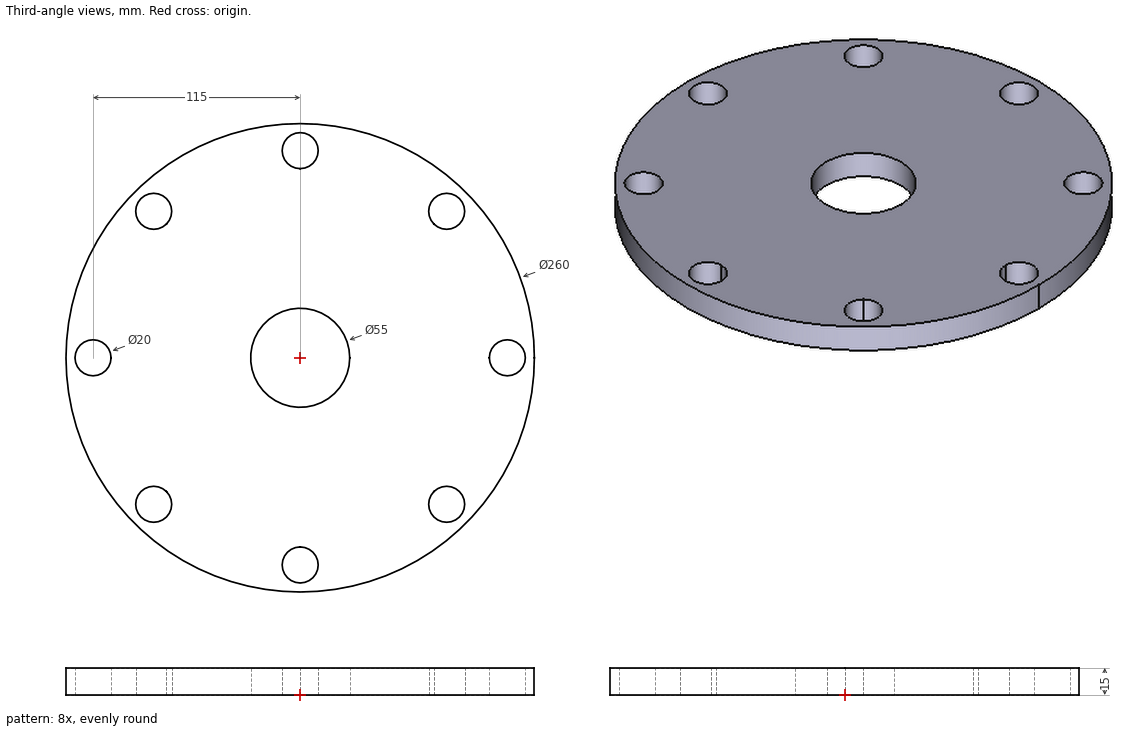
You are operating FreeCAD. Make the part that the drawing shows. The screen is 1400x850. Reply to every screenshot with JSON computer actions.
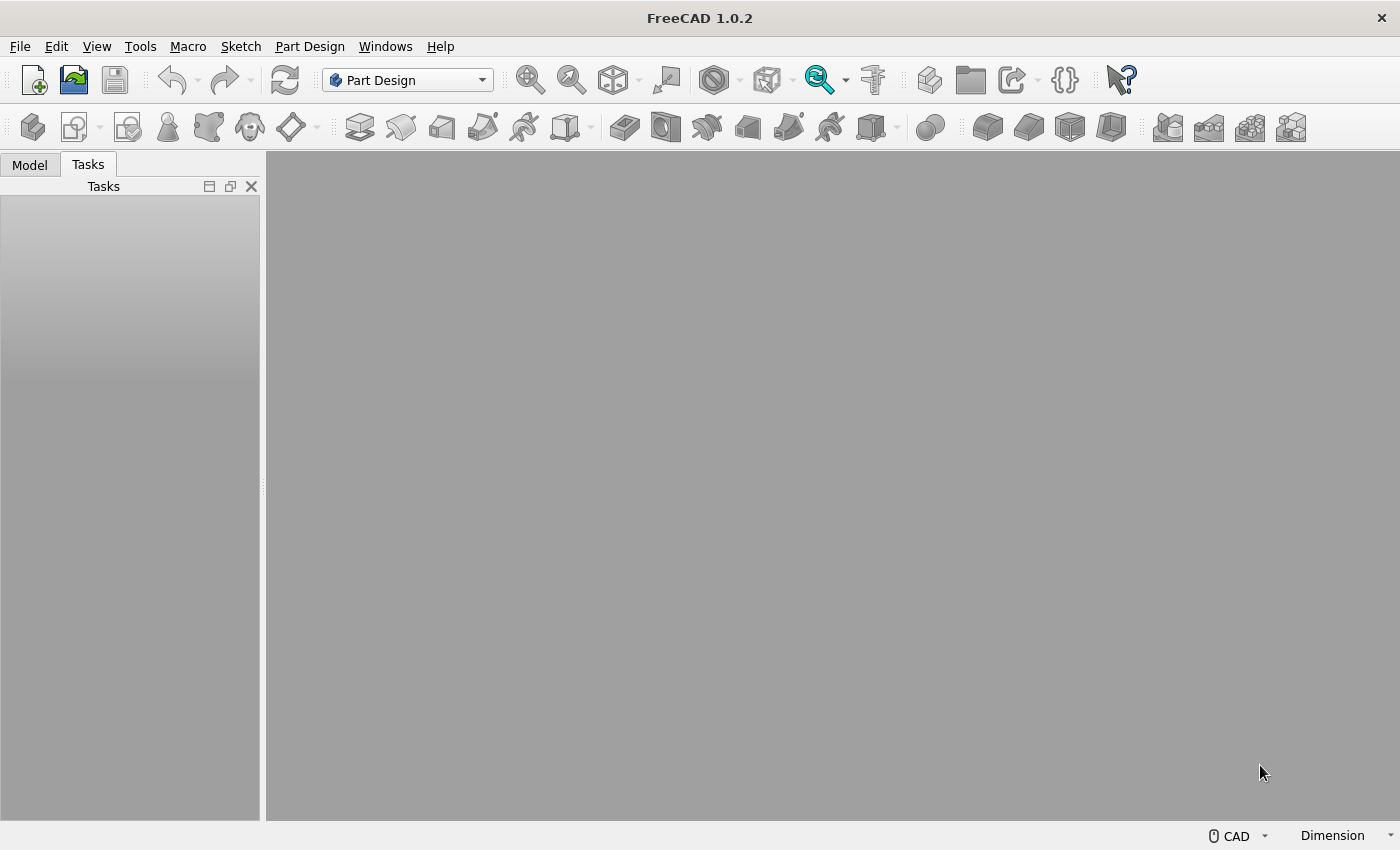
{"action": "left_click", "coordinate": [33, 80]}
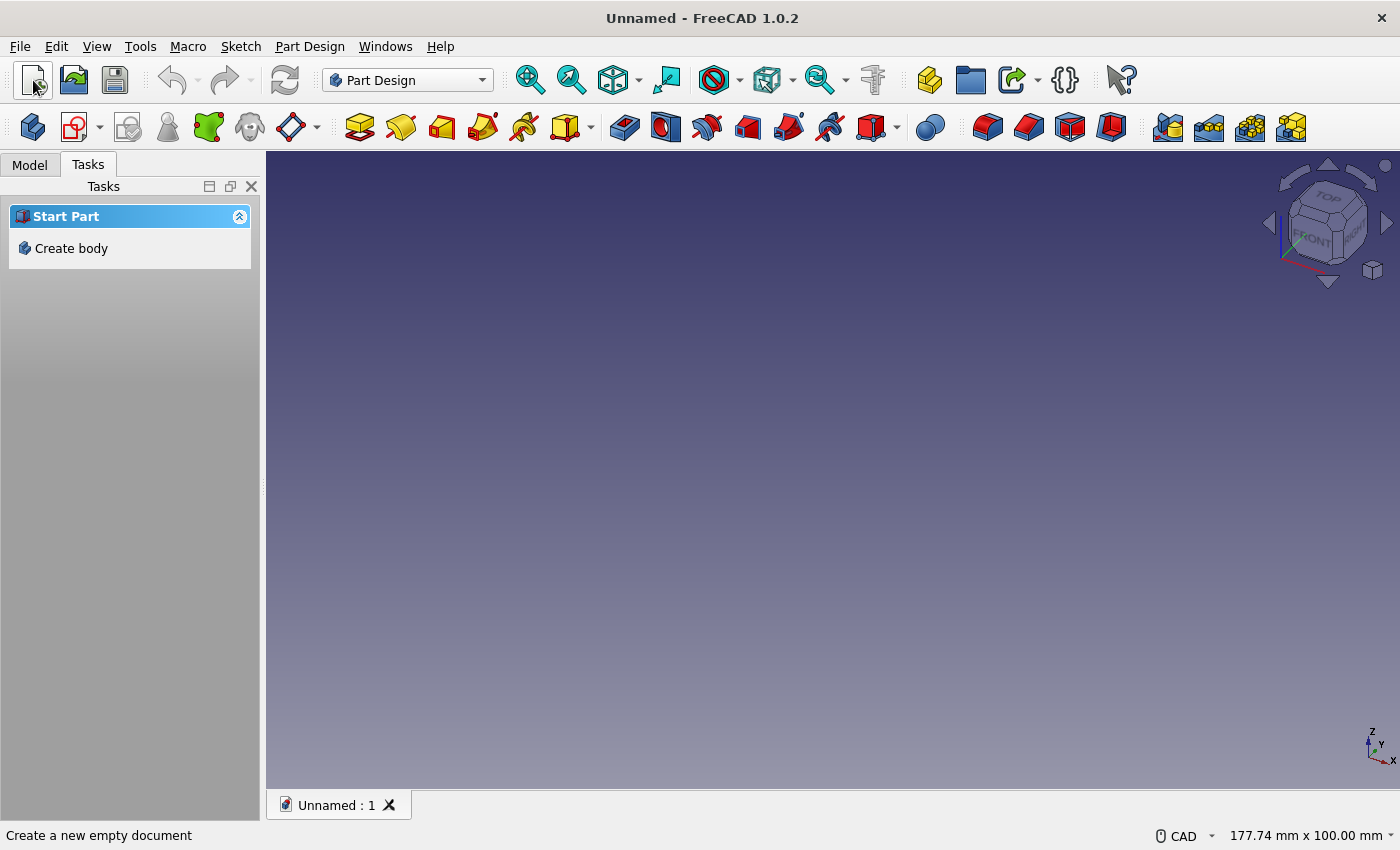
{"action": "left_click", "coordinate": [74, 128]}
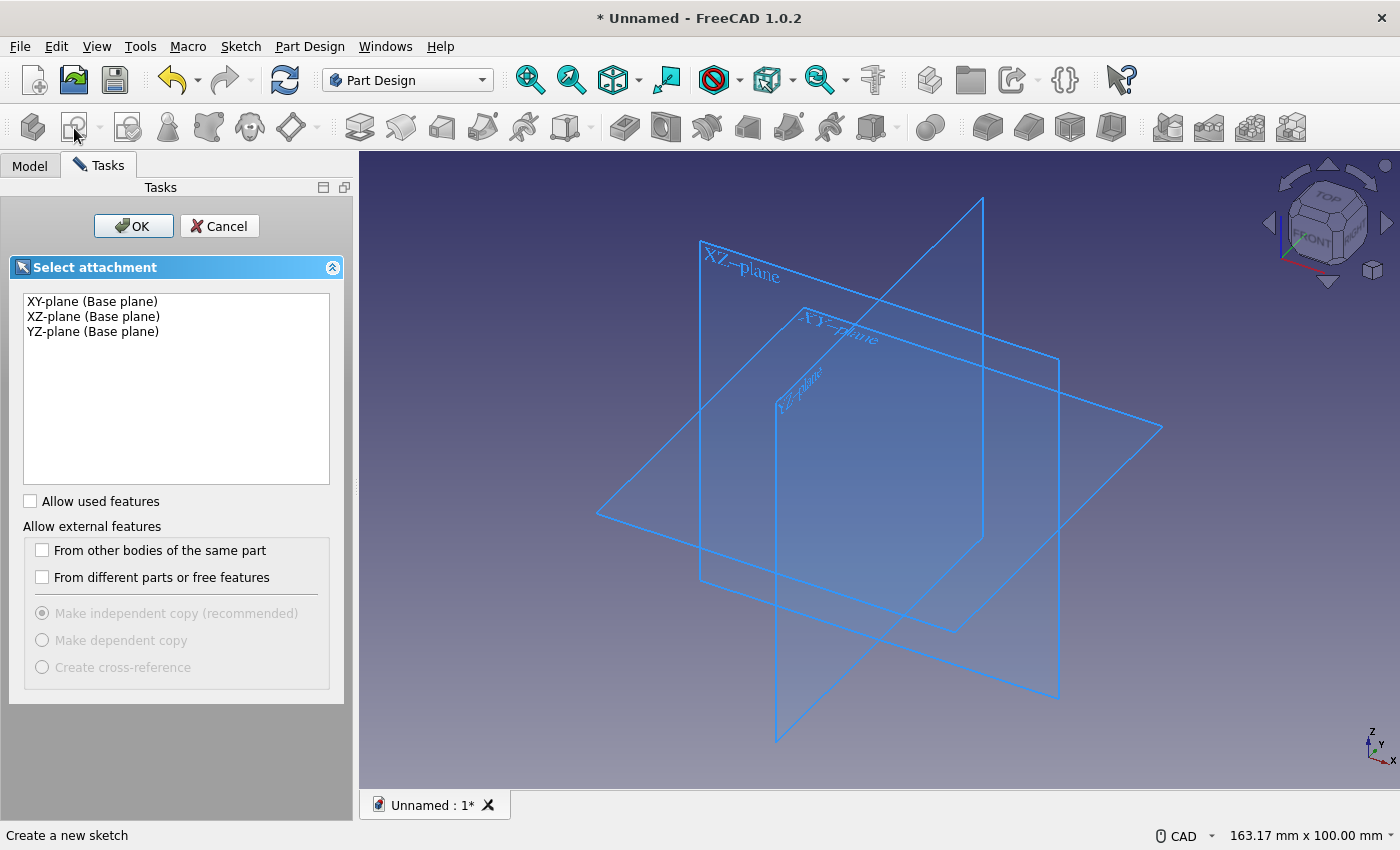
{"action": "left_click", "coordinate": [84, 302]}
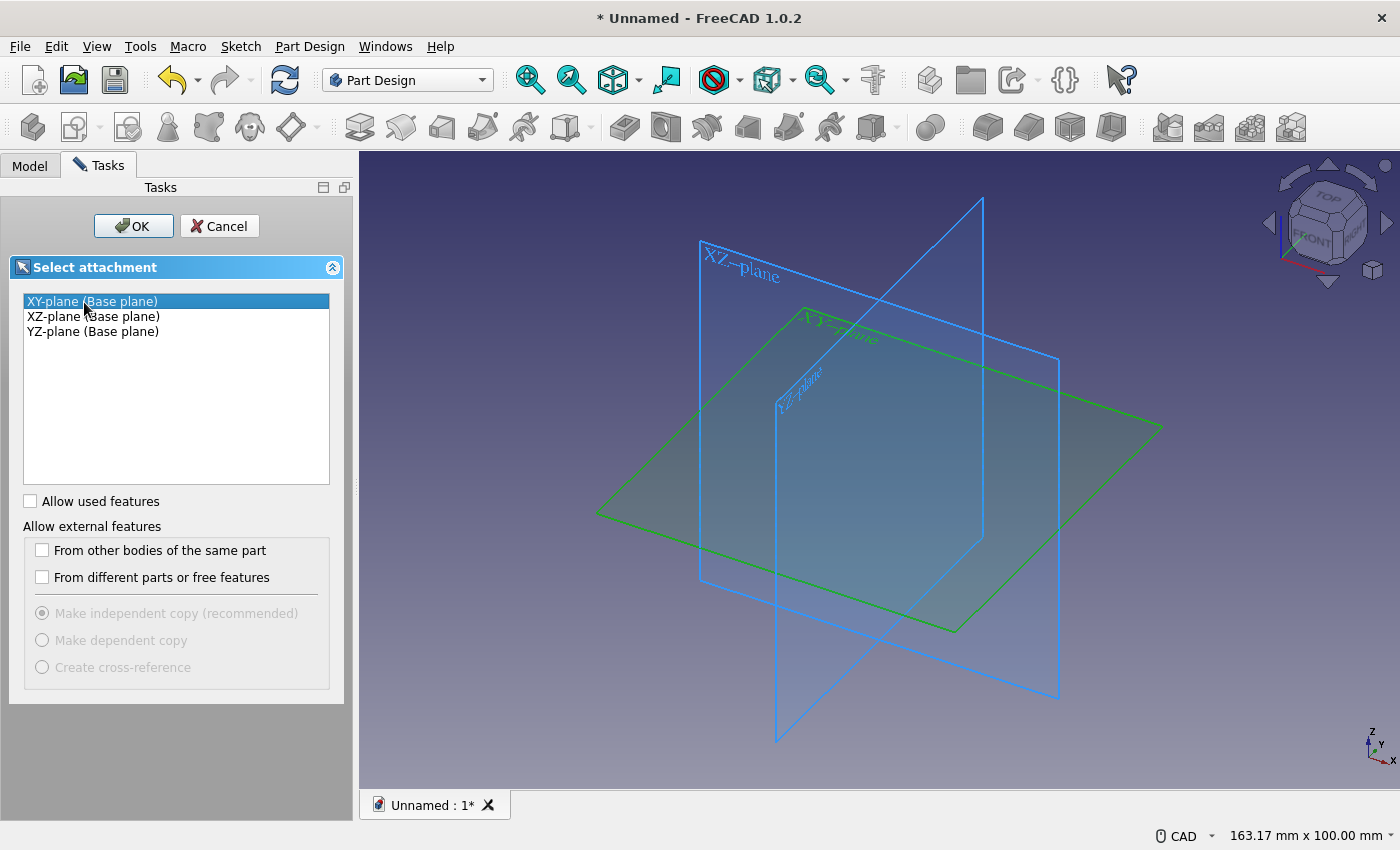
{"action": "left_click", "coordinate": [134, 226]}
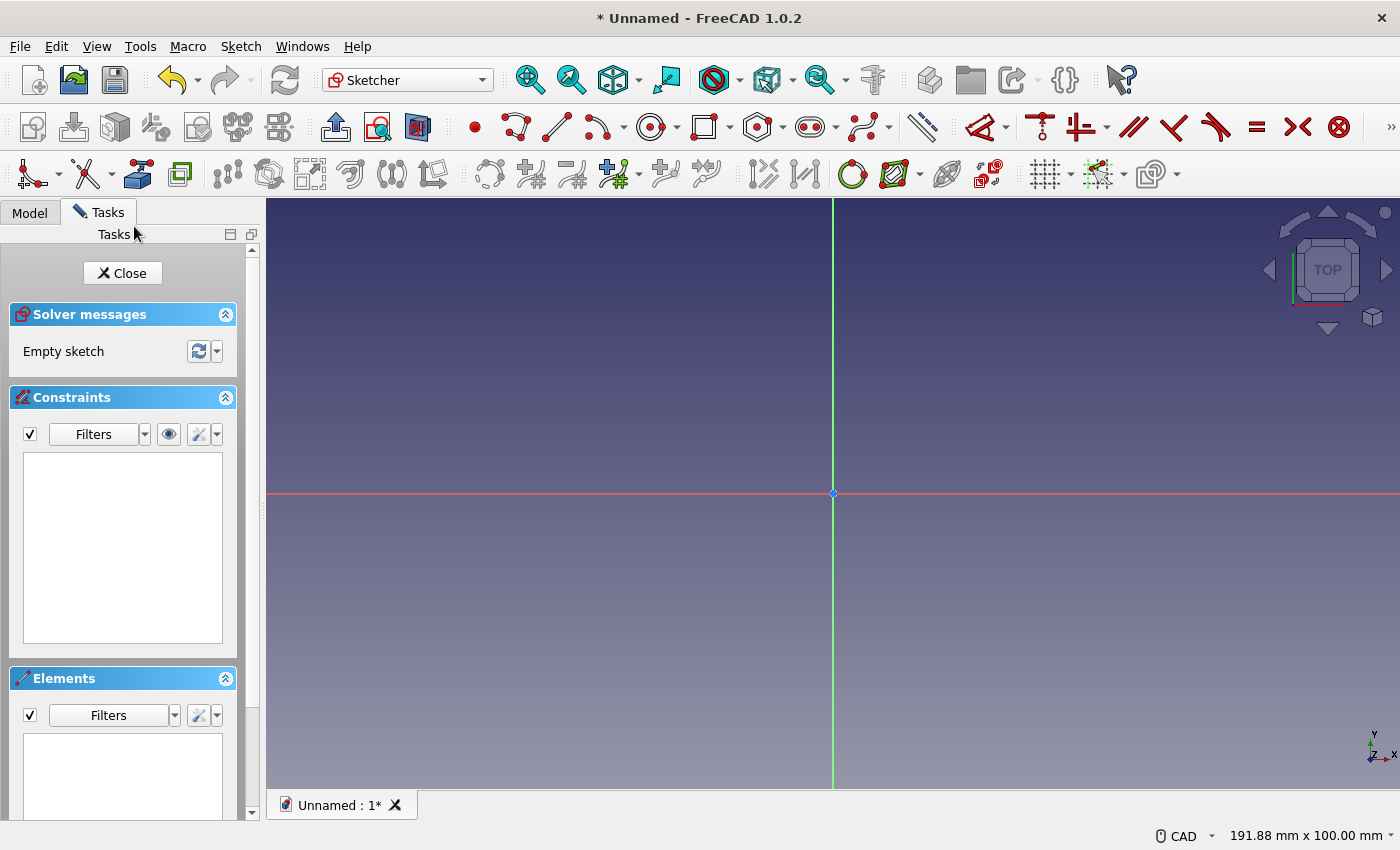
{"action": "scroll", "coordinate": [742, 494], "scroll_direction": "down", "scroll_amount": 7}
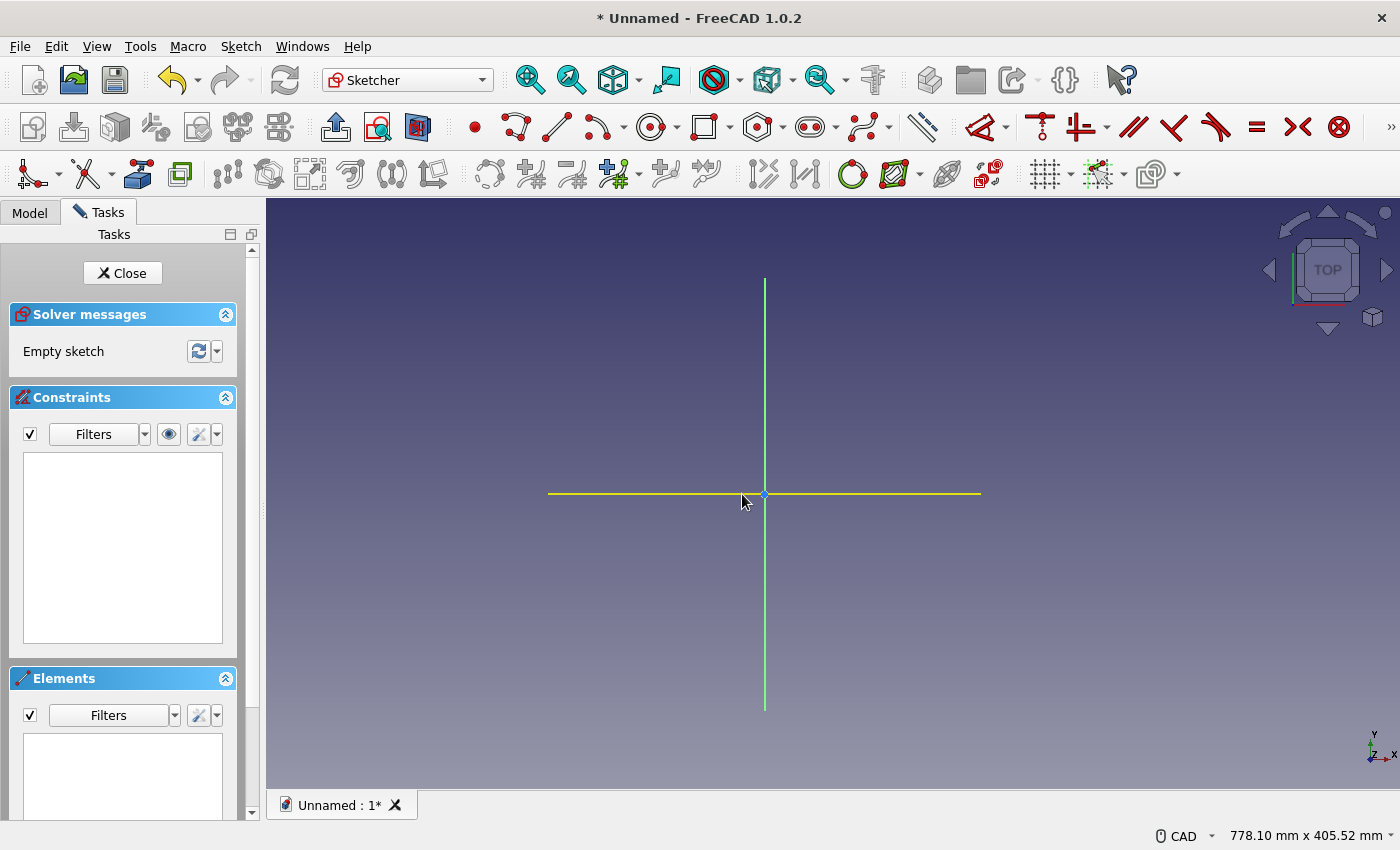
{"action": "left_click", "coordinate": [650, 128]}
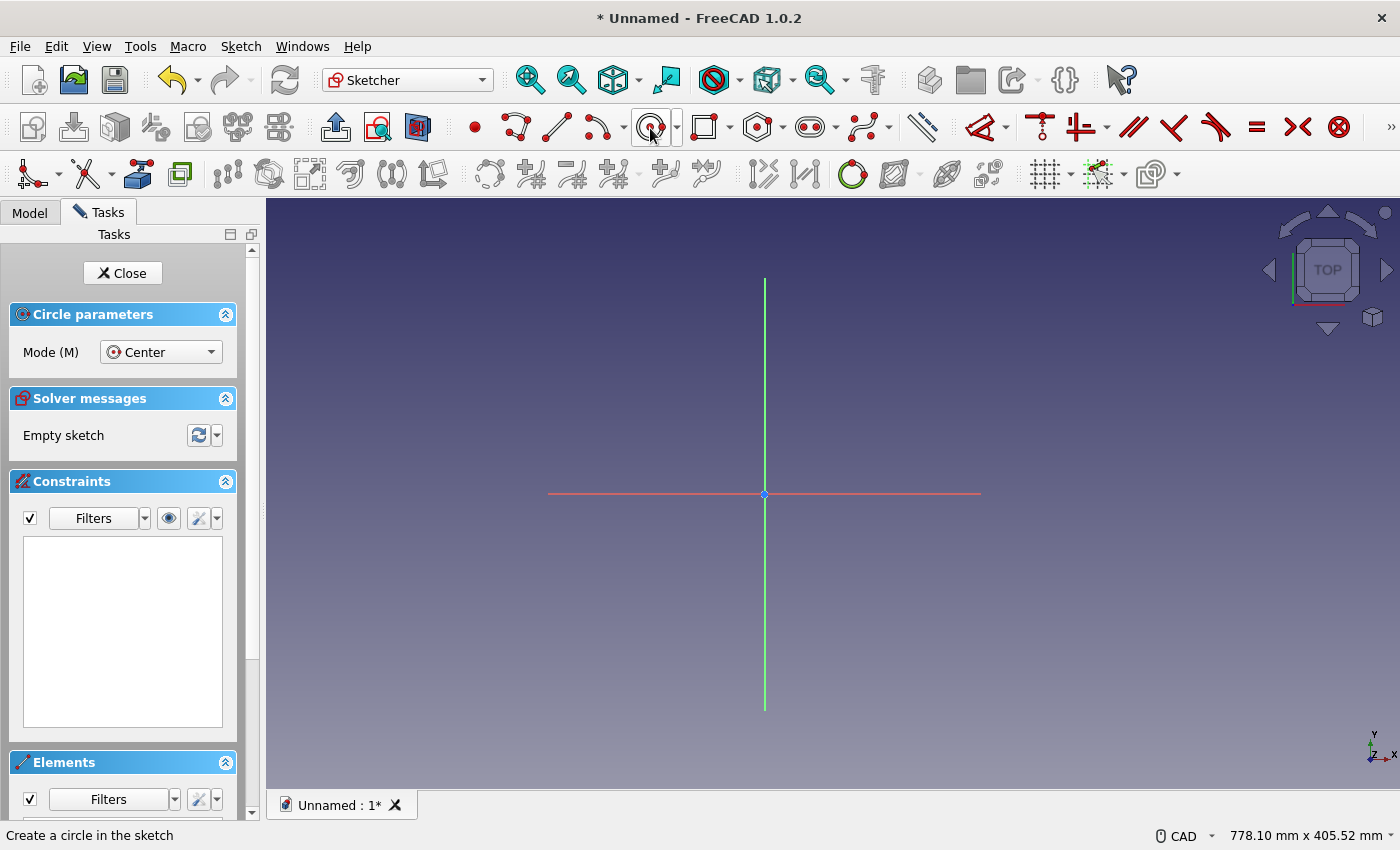
{"action": "left_click", "coordinate": [765, 494]}
{"action": "left_click", "coordinate": [899, 360]}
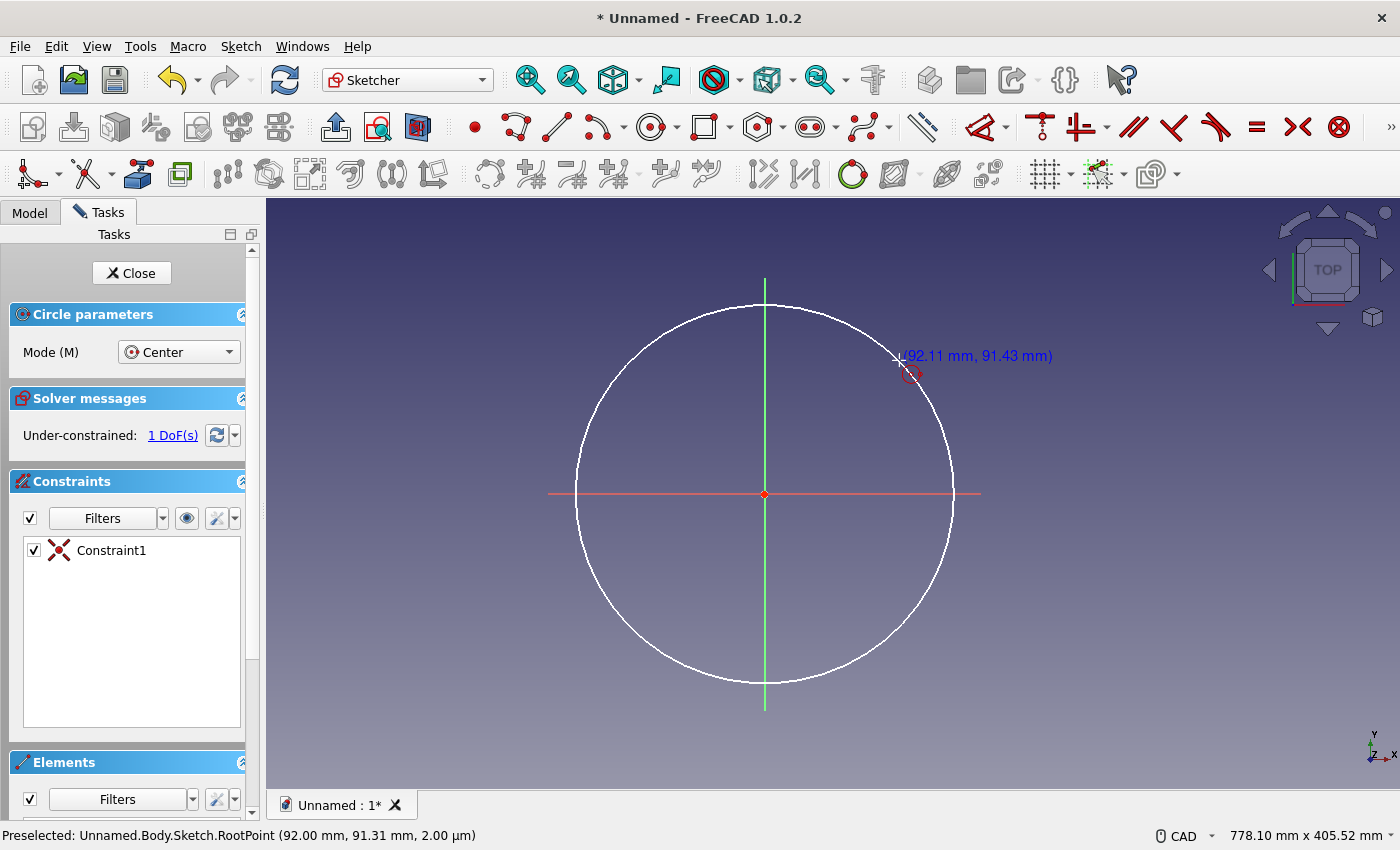
{"action": "left_click", "coordinate": [765, 494]}
{"action": "left_click", "coordinate": [793, 466]}
{"action": "key", "text": "Escape"}